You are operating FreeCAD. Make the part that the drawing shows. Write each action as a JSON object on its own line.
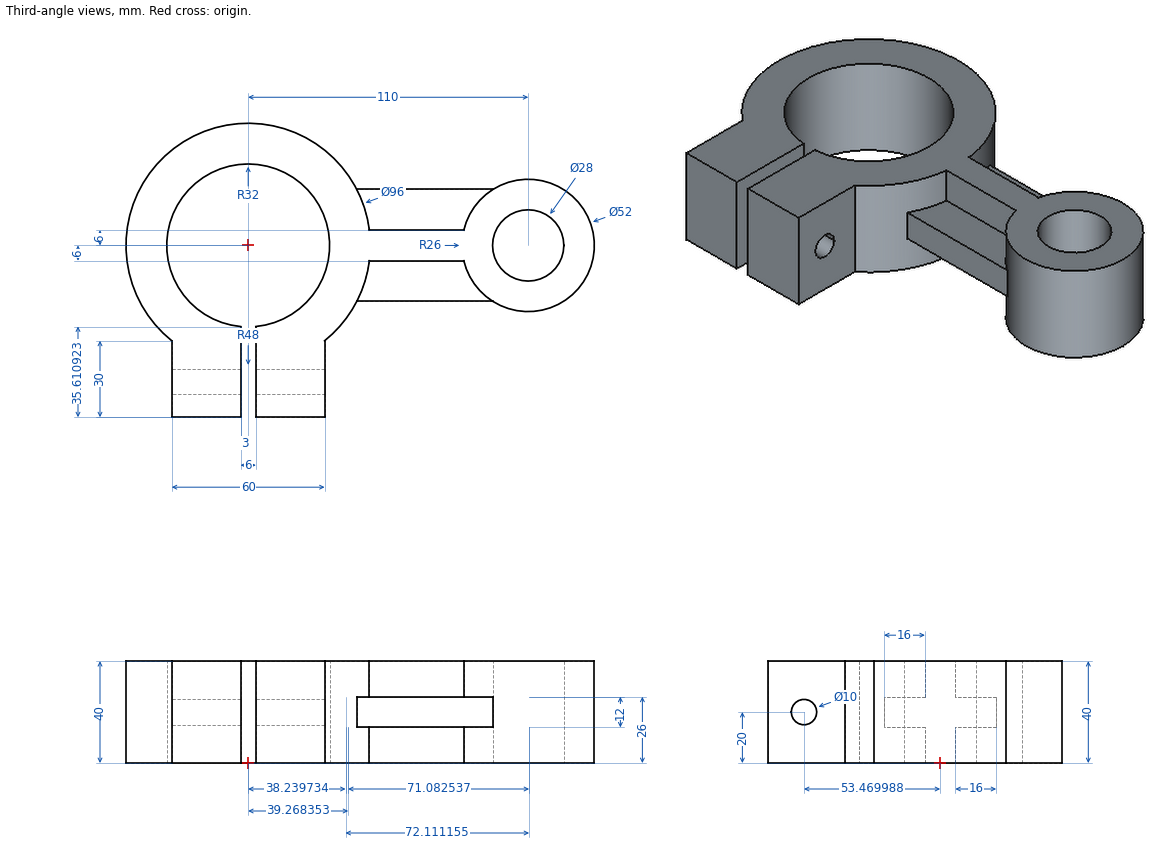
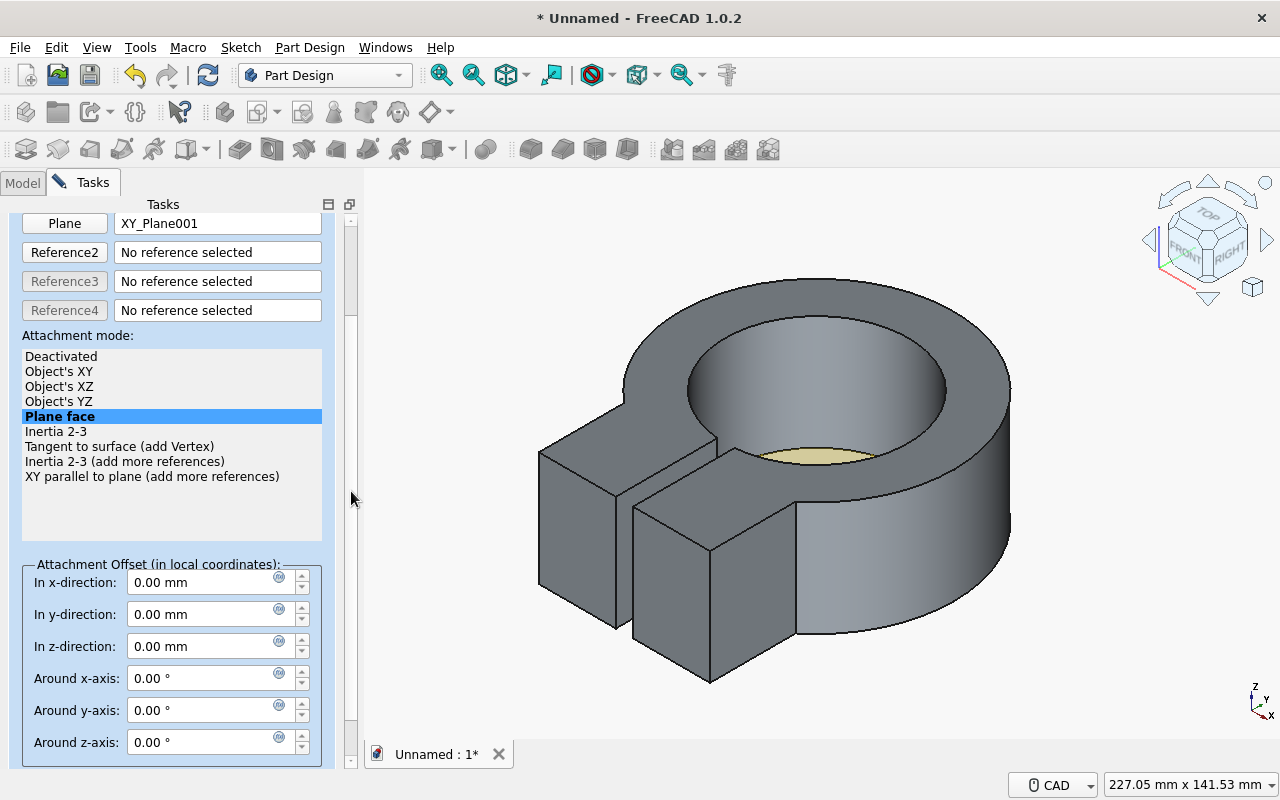
{"action": "triple_click", "coordinate": [210, 646]}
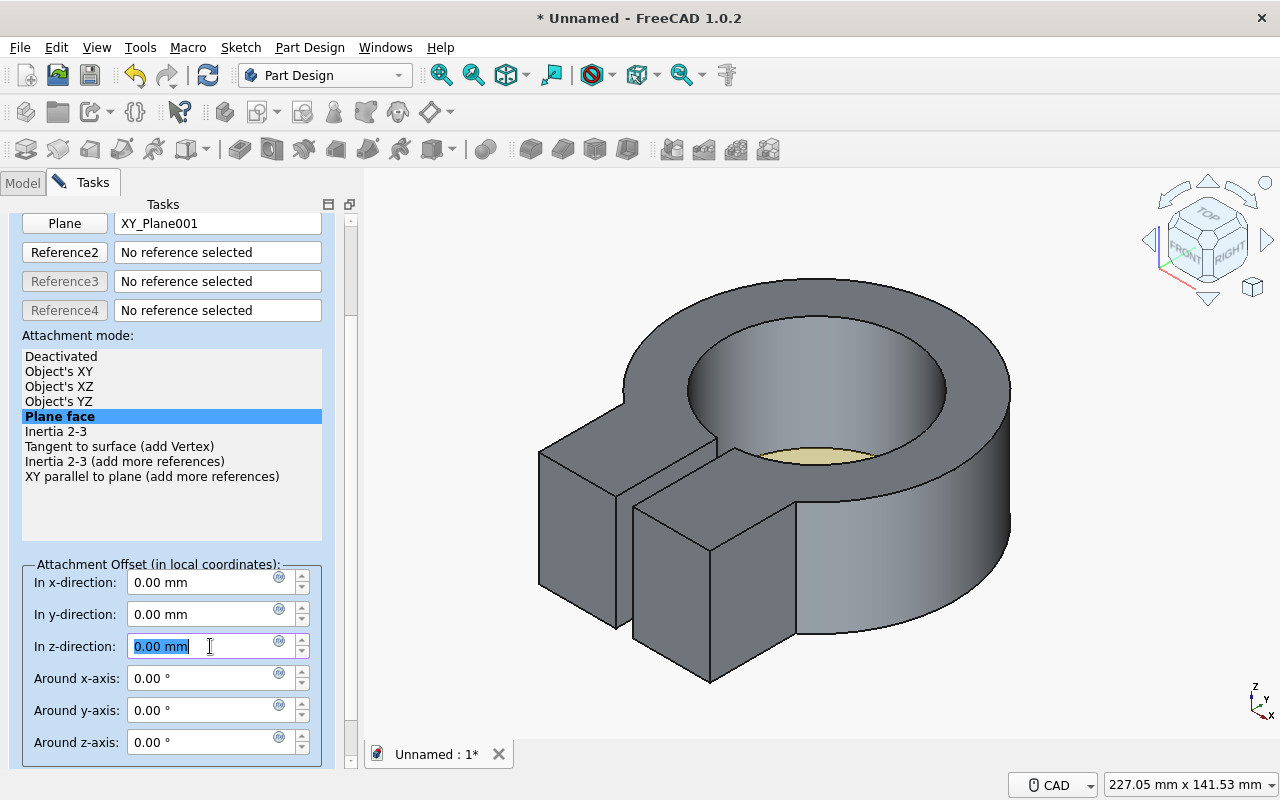
{"action": "type", "text": "40"}
{"action": "key", "text": "Tab"}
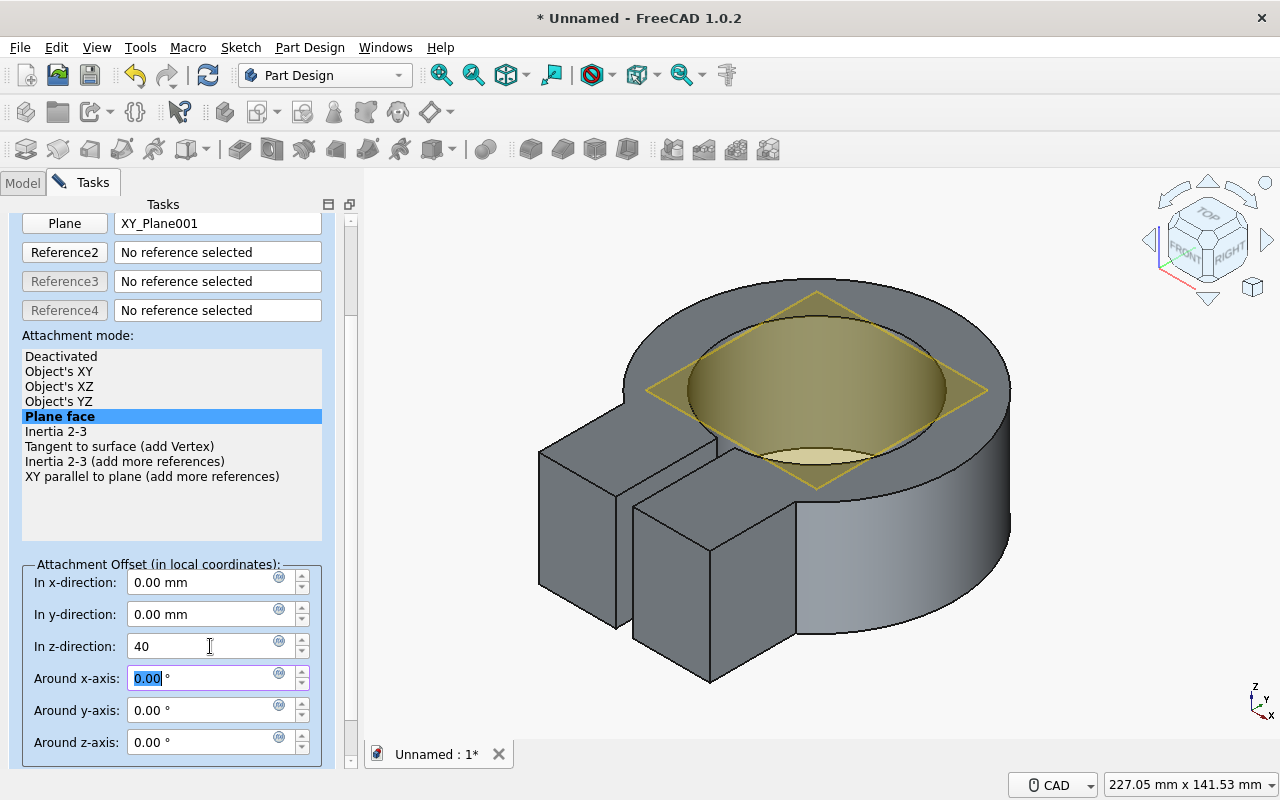
{"action": "scroll", "coordinate": [351, 491], "scroll_direction": "up", "scroll_amount": 3}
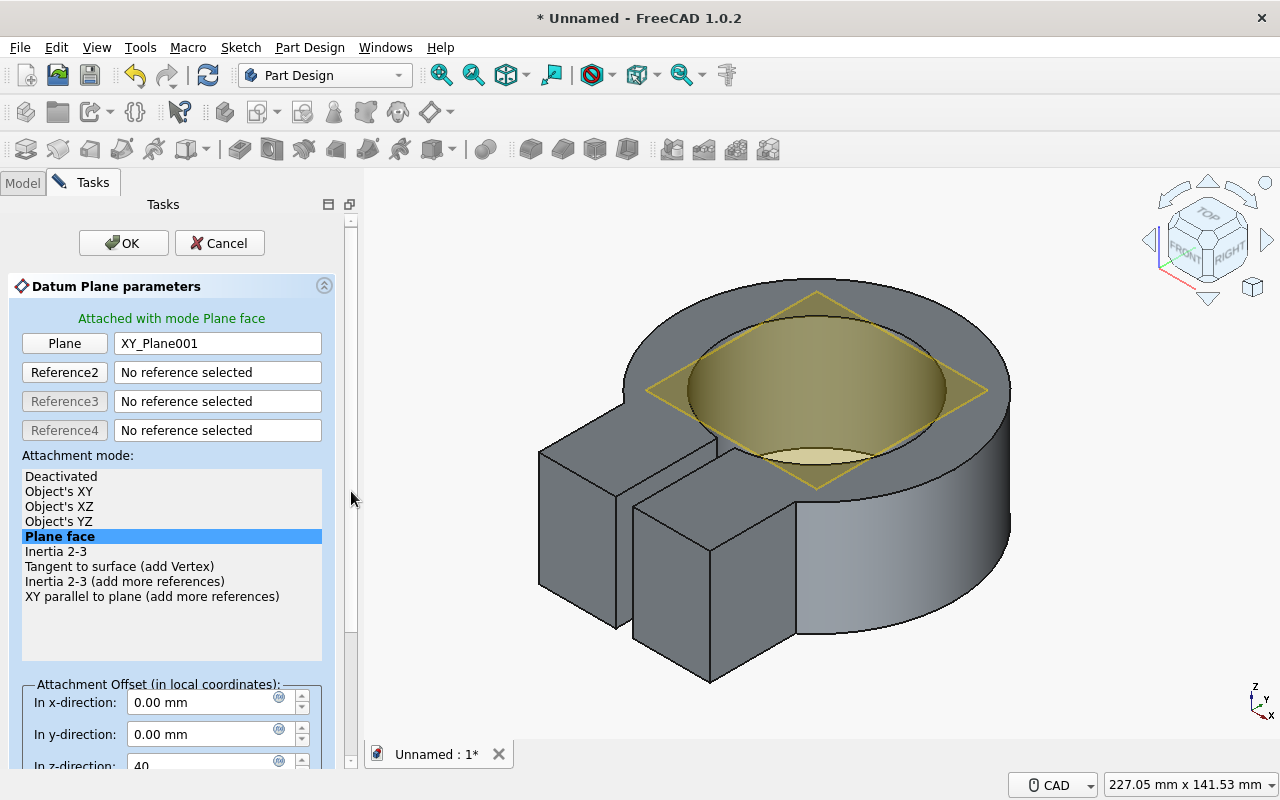
{"action": "left_click", "coordinate": [124, 243]}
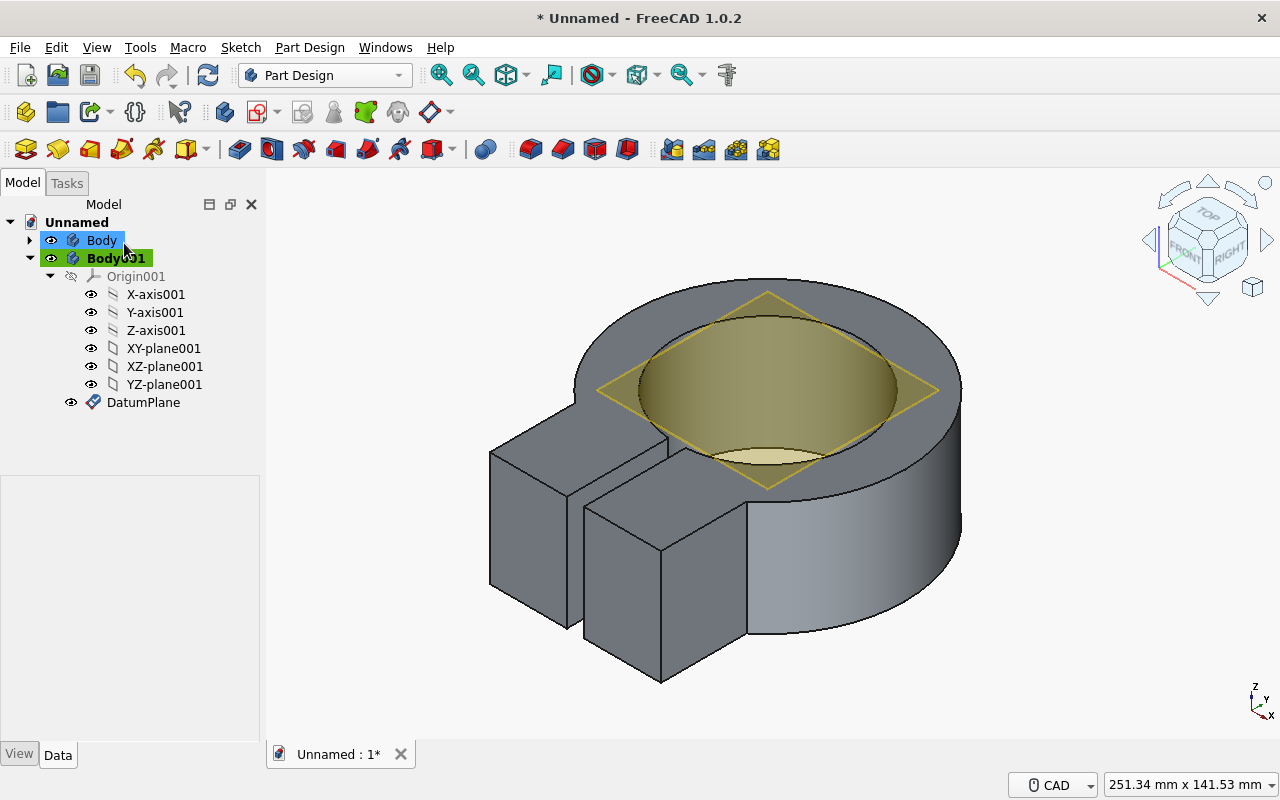
{"action": "left_click", "coordinate": [116, 402]}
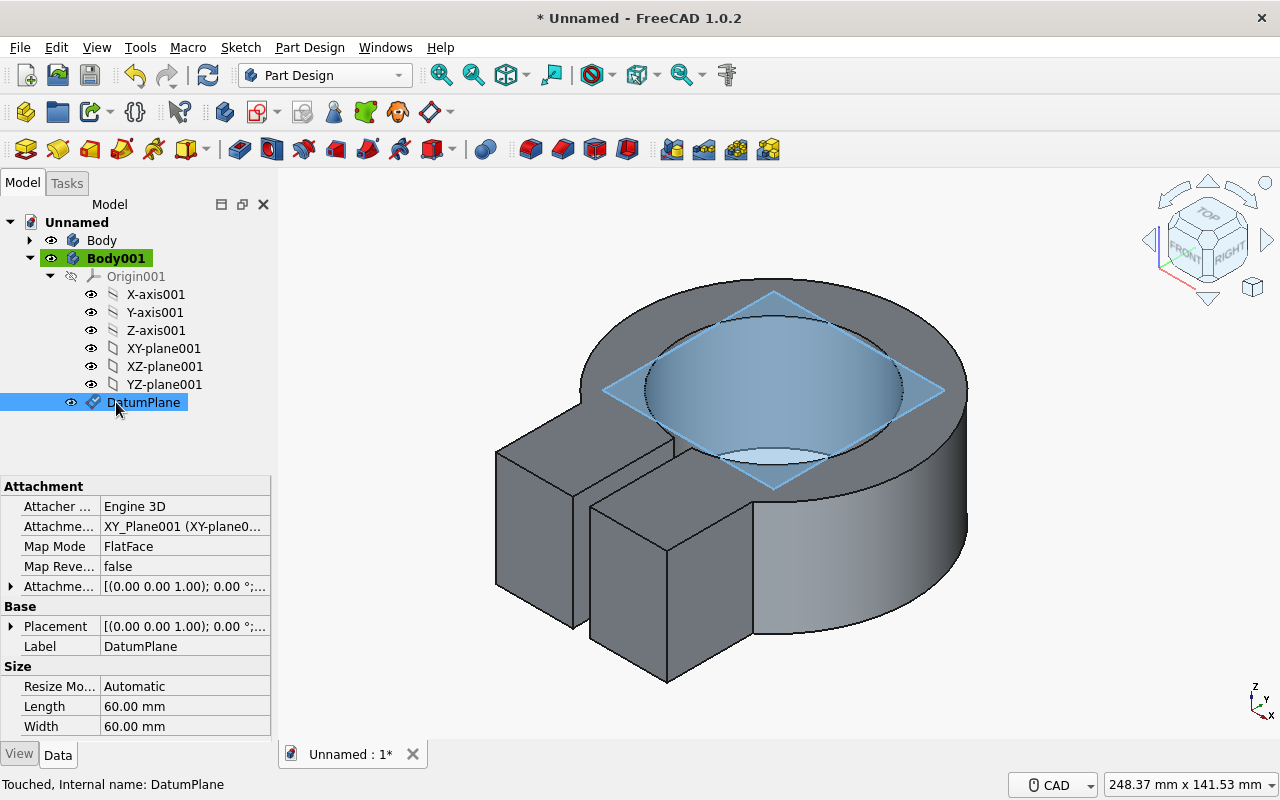
{"action": "left_click", "coordinate": [258, 112]}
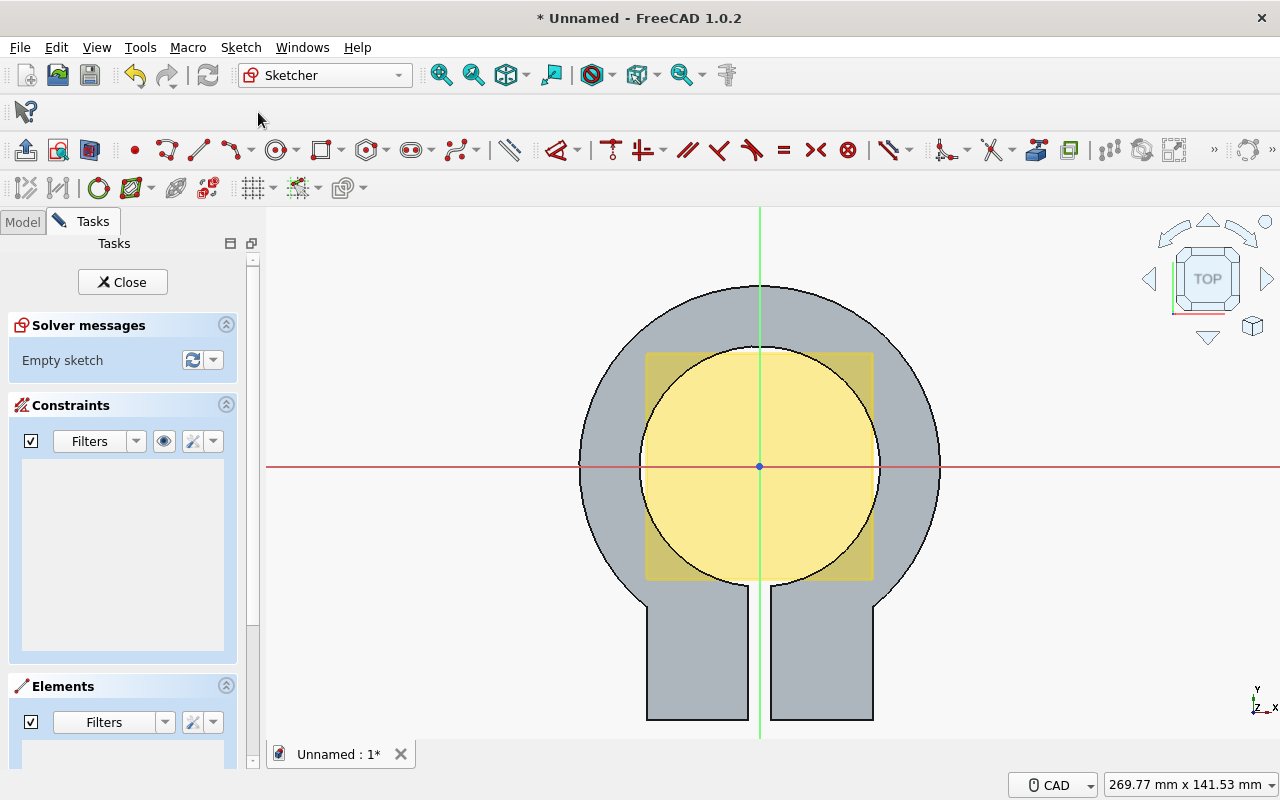
{"action": "scroll", "coordinate": [704, 473], "scroll_direction": "down", "scroll_amount": 5}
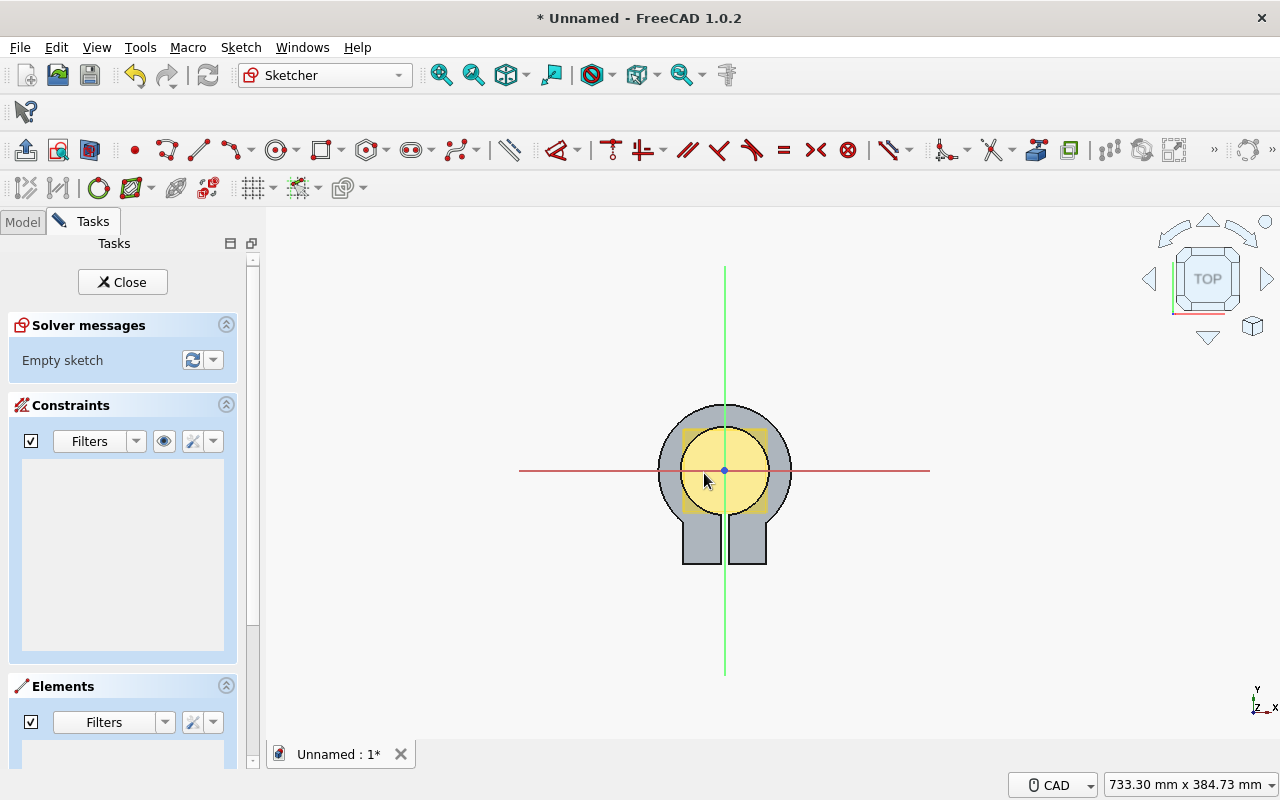
{"action": "scroll", "coordinate": [921, 470], "scroll_direction": "up", "scroll_amount": 8}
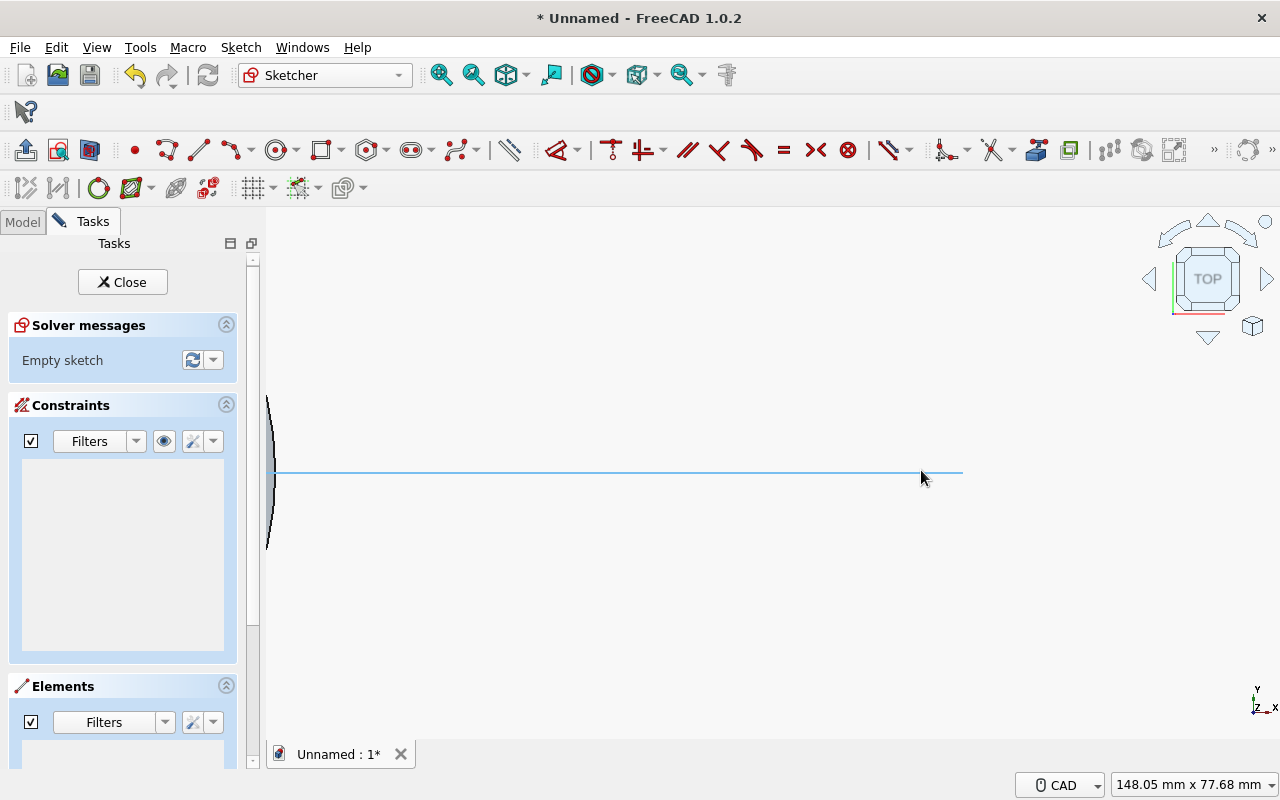
{"action": "left_click", "coordinate": [276, 150]}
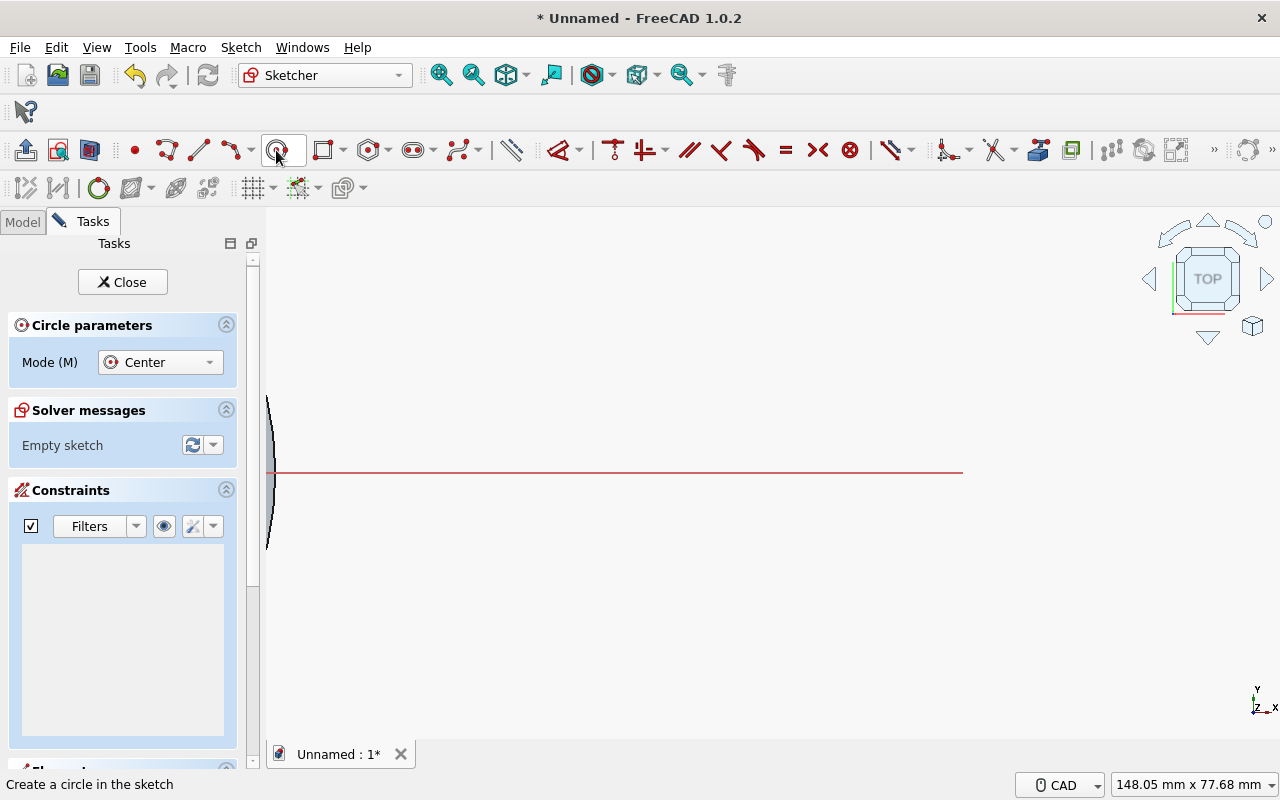
{"action": "left_click", "coordinate": [700, 473]}
{"action": "left_click", "coordinate": [826, 347]}
{"action": "key", "text": "Escape"}